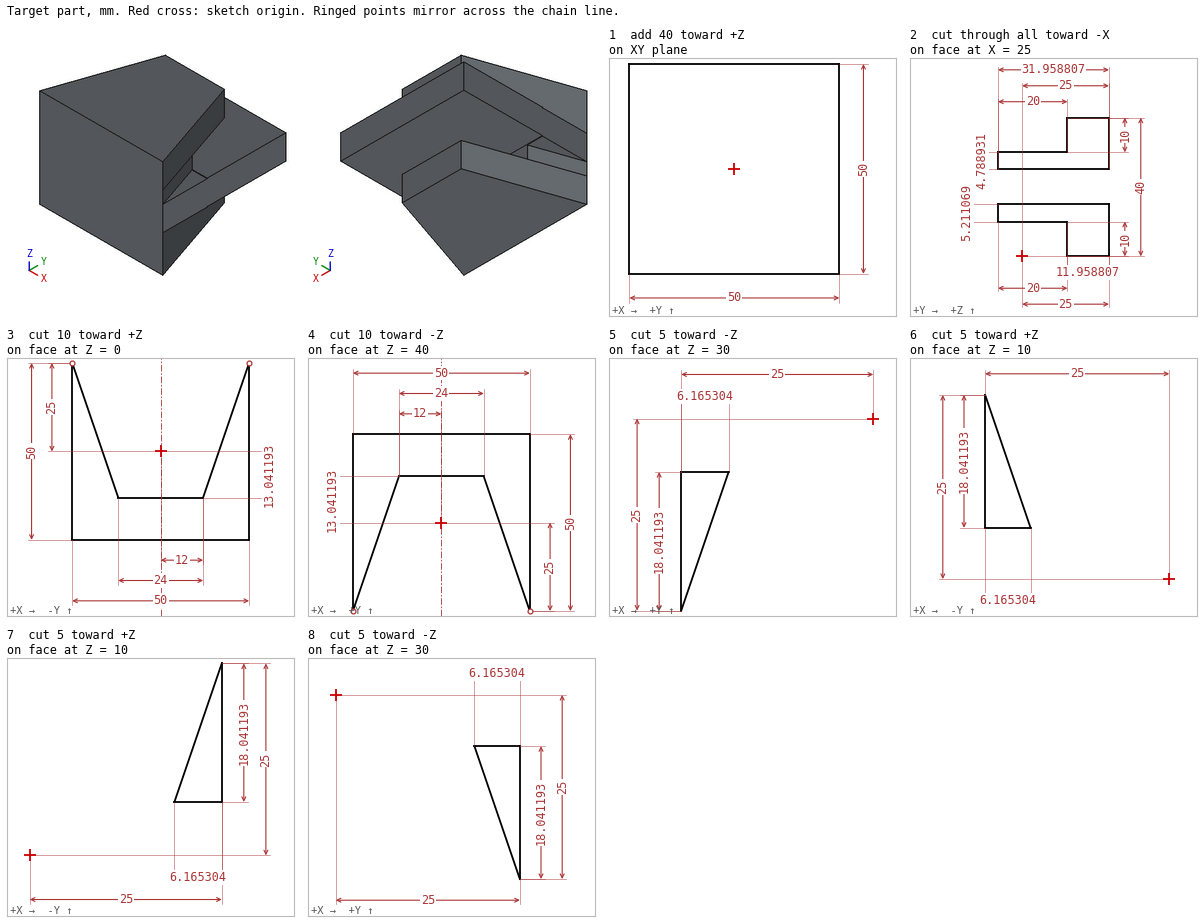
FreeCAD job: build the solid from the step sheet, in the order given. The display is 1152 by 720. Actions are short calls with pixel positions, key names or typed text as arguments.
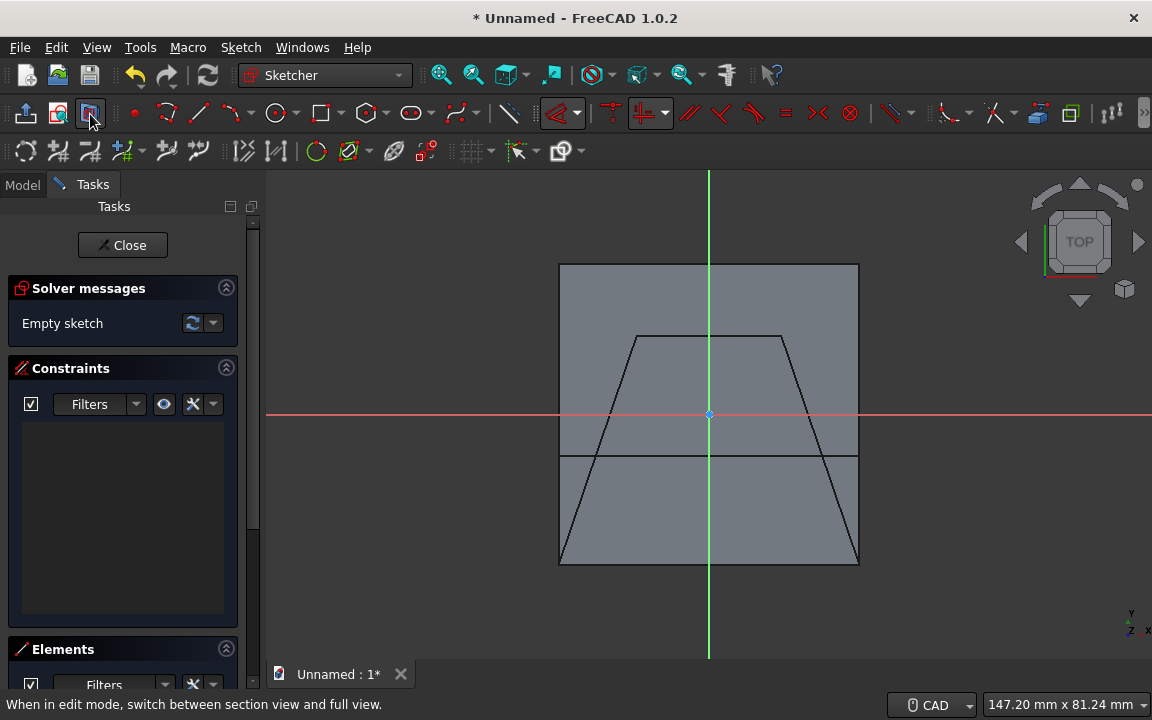
scroll(628, 551, up, 4)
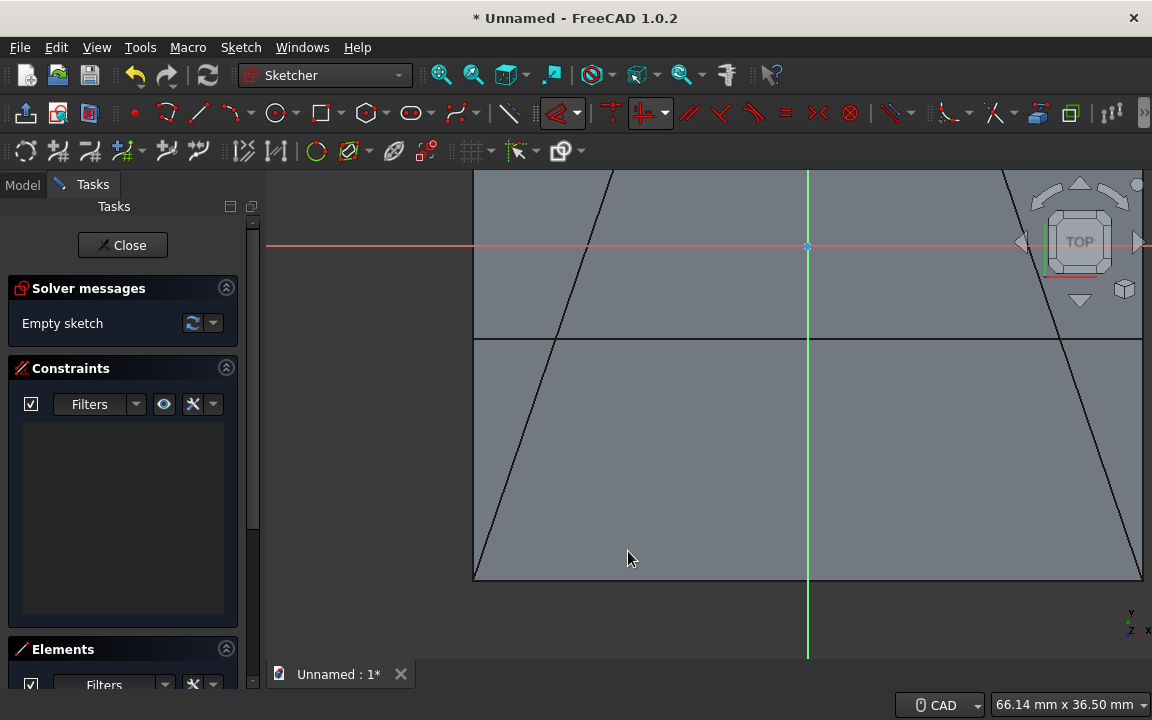
key(g)
key(m)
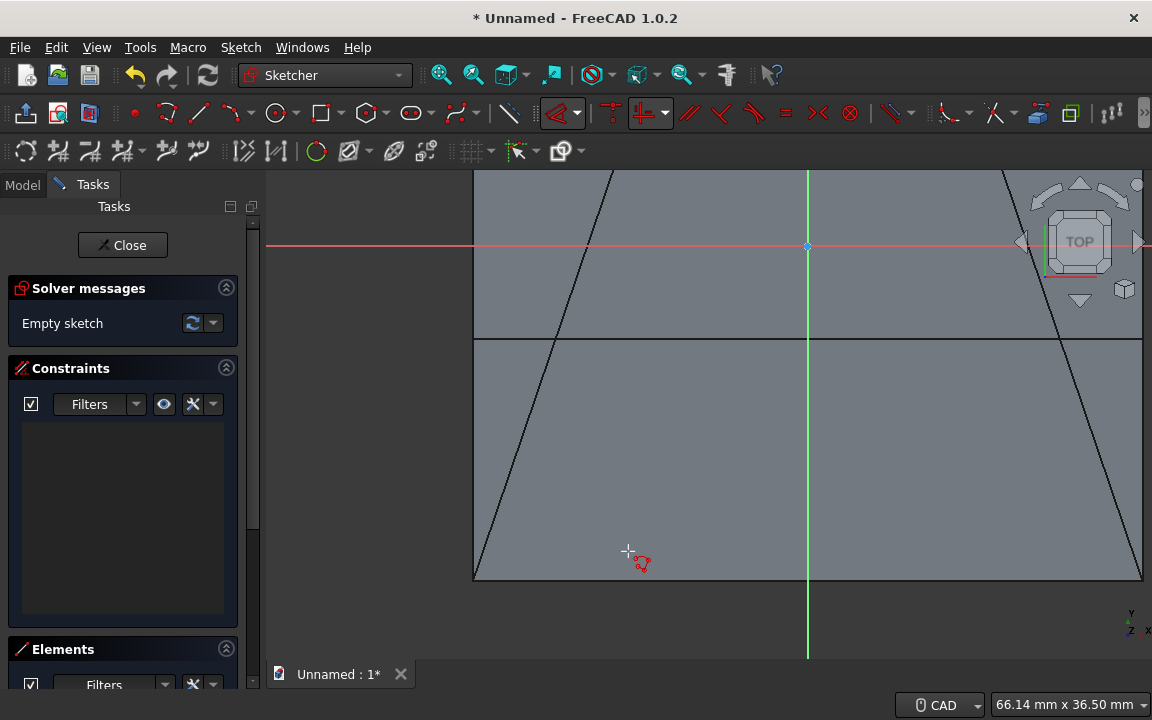
click(555, 339)
click(473, 339)
click(473, 581)
click(555, 340)
key(Escape)
key(Escape)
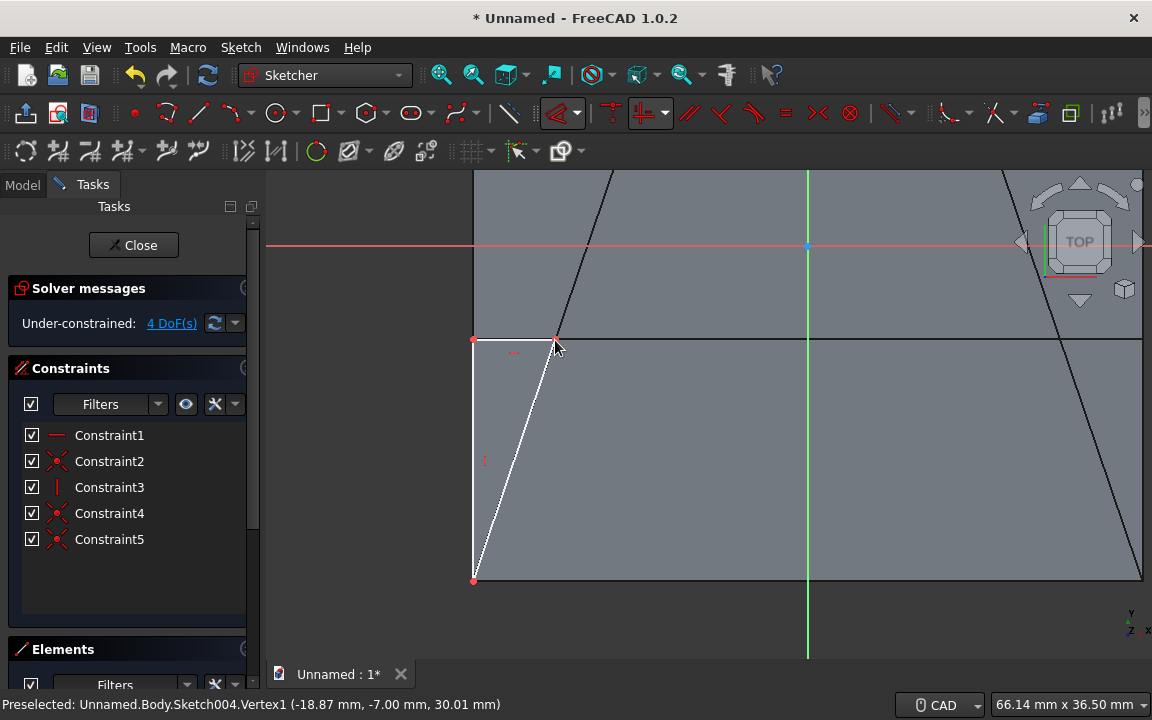
click(473, 340)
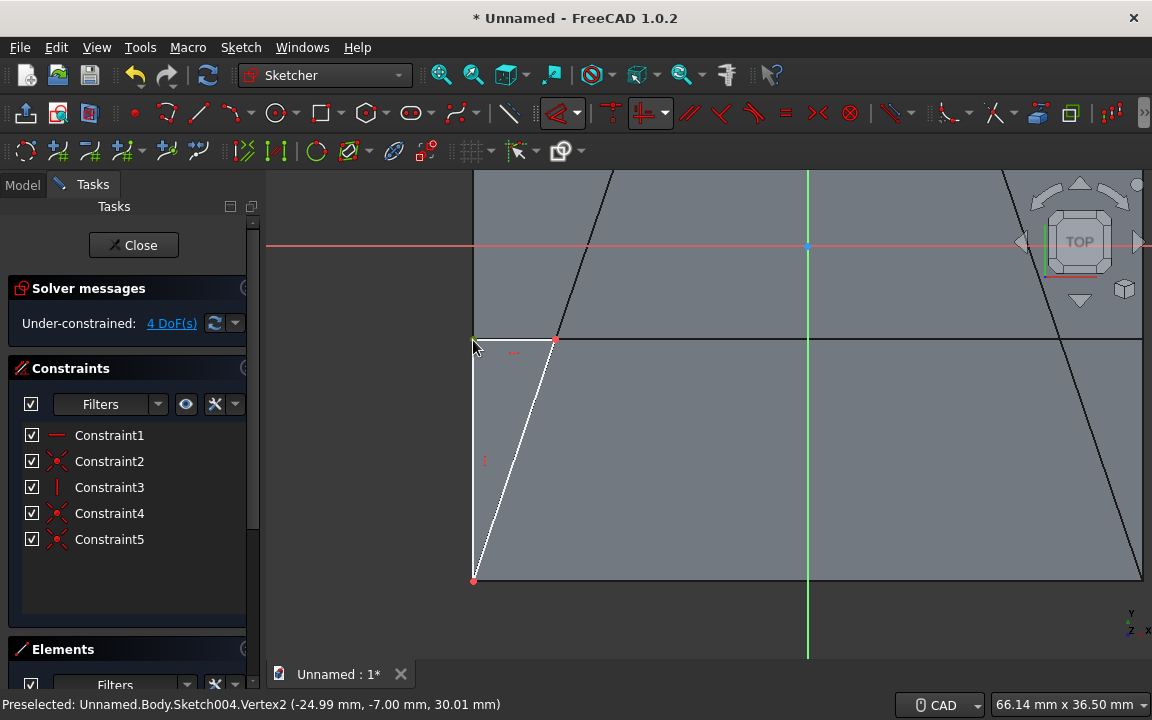
key(l)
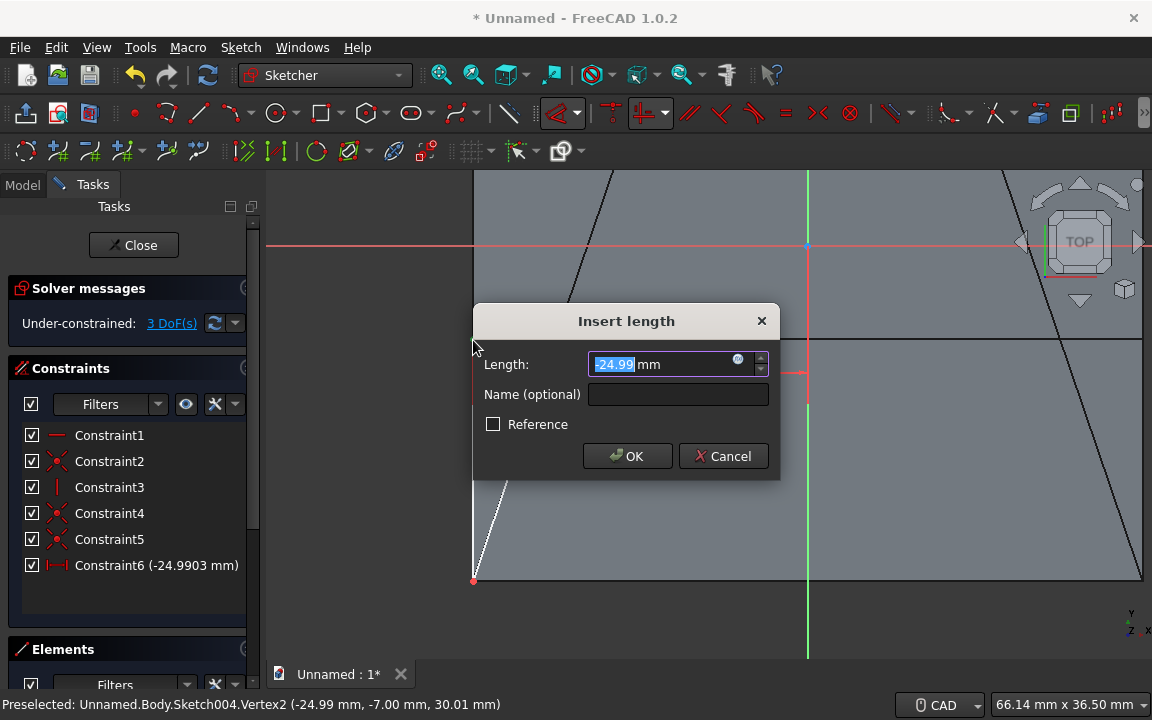
text(-25)
key(Return)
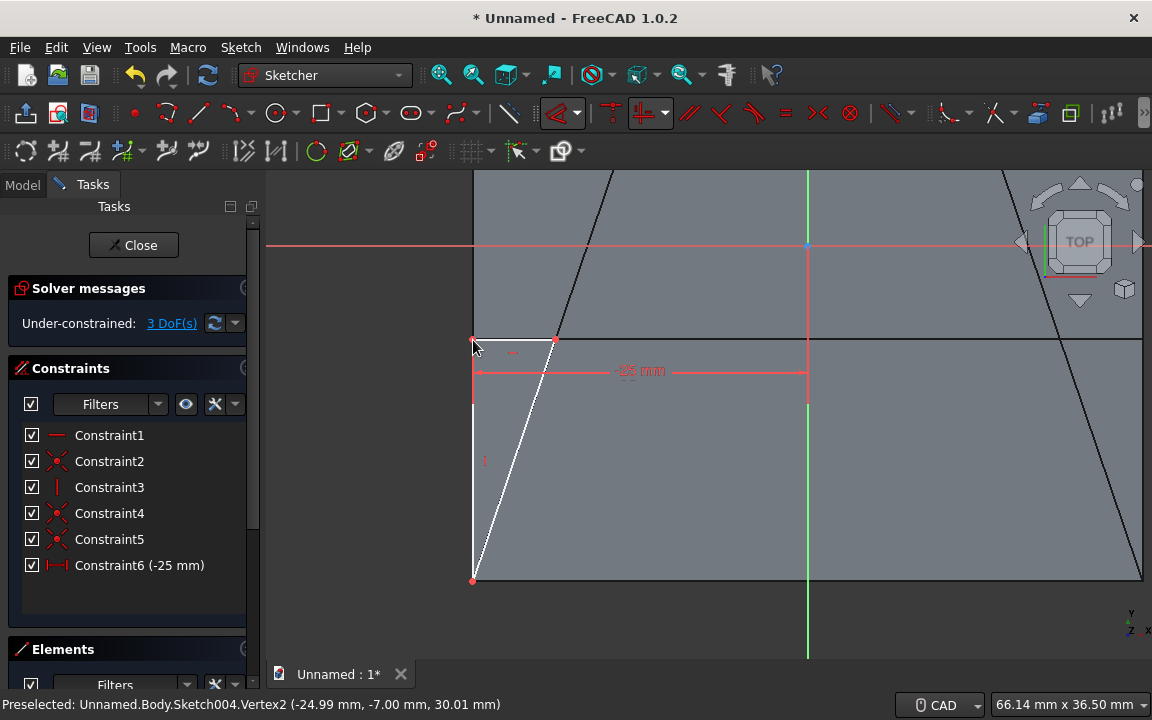
click(473, 582)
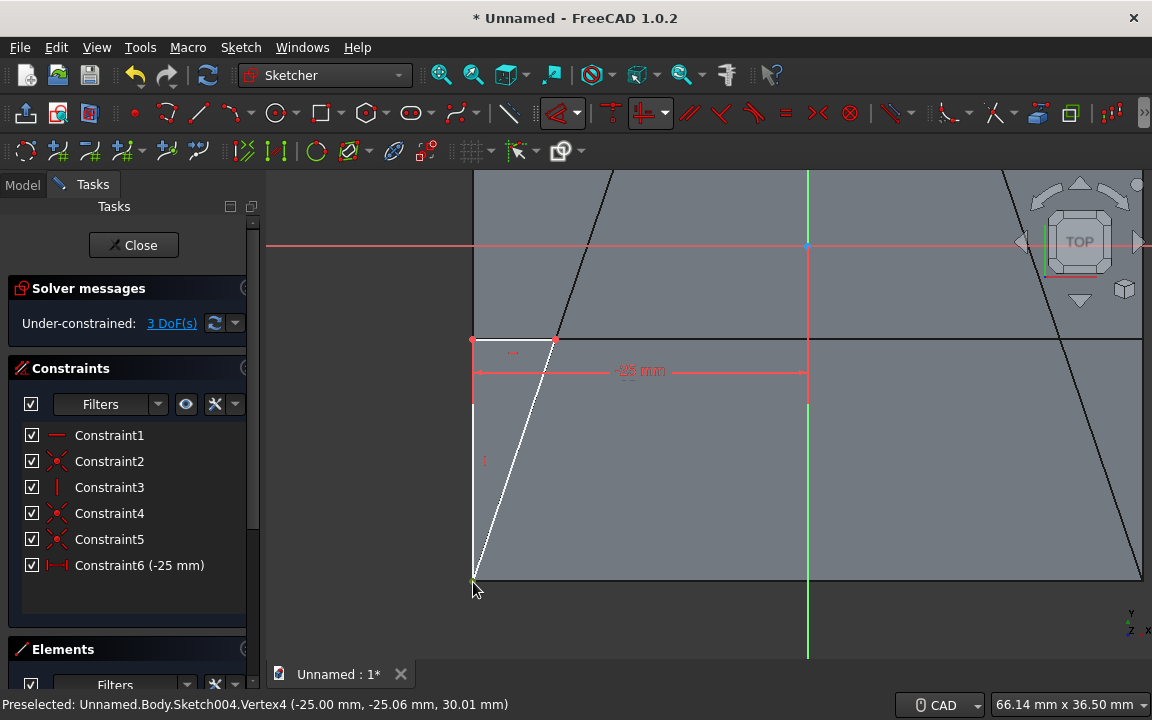
click(580, 114)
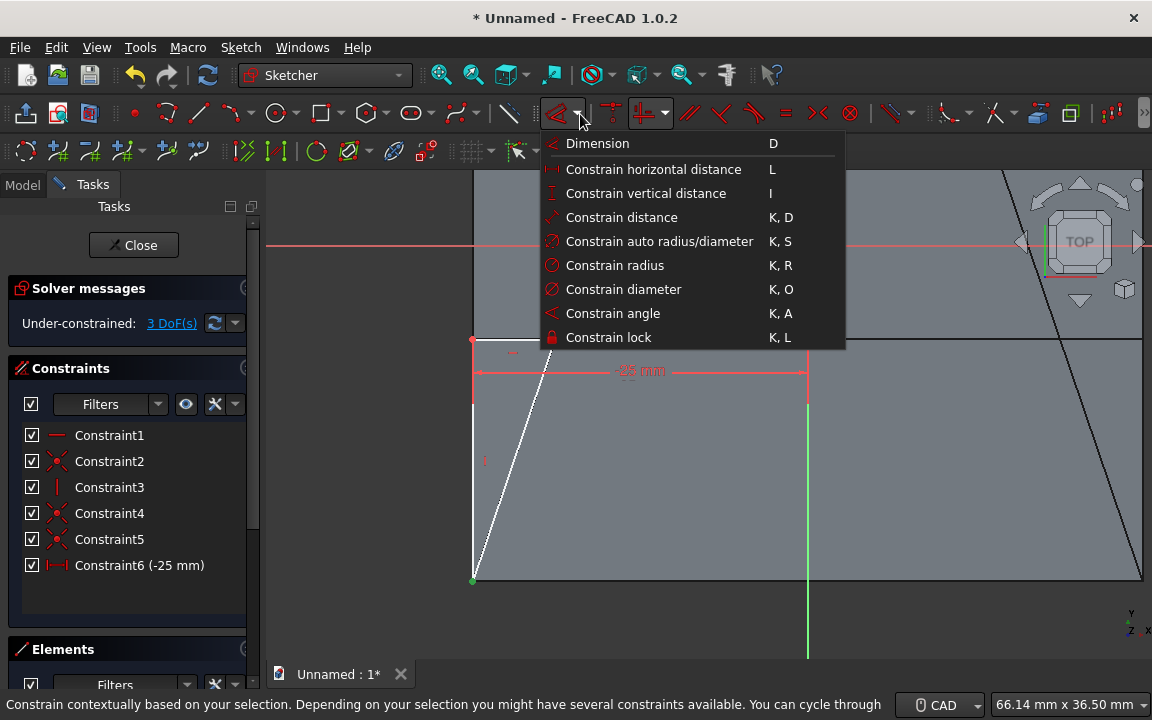
click(693, 193)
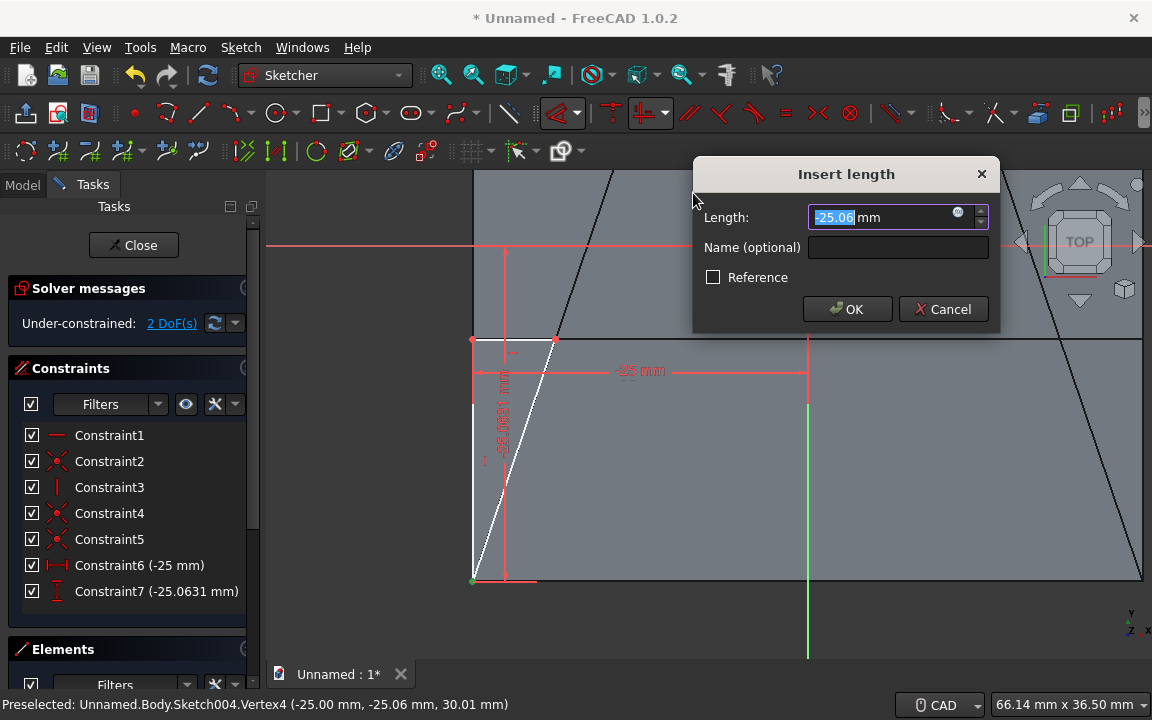
text(-25)
key(Return)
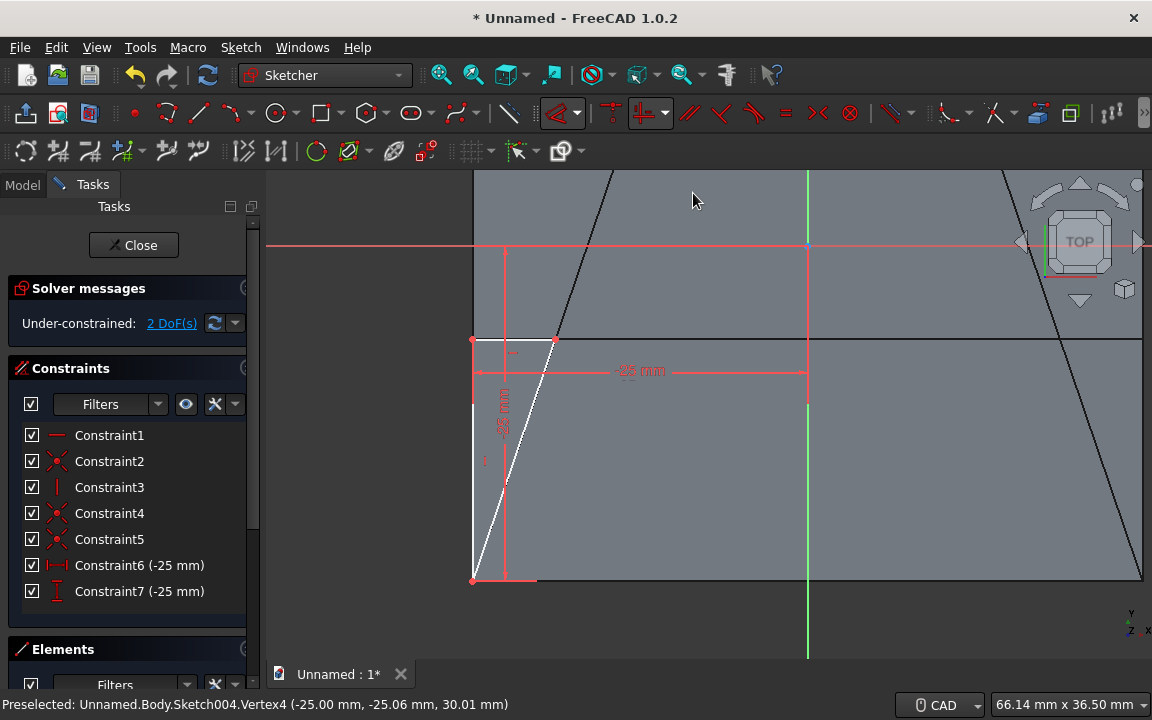
click(530, 340)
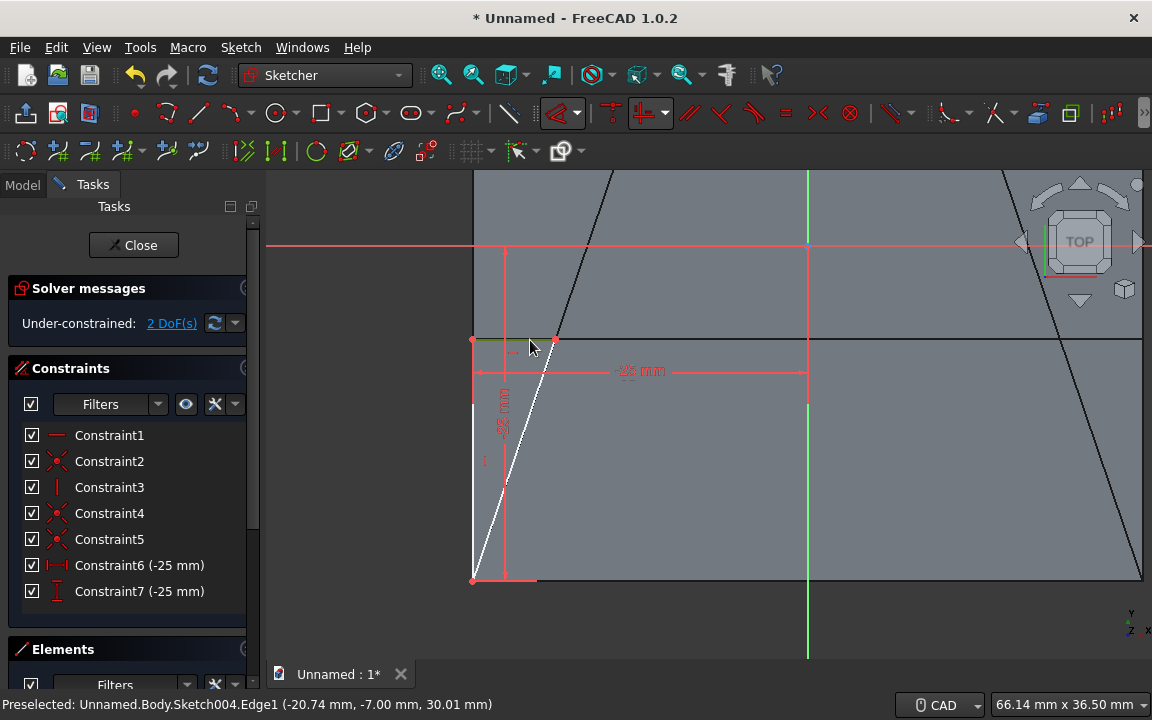
key(l)